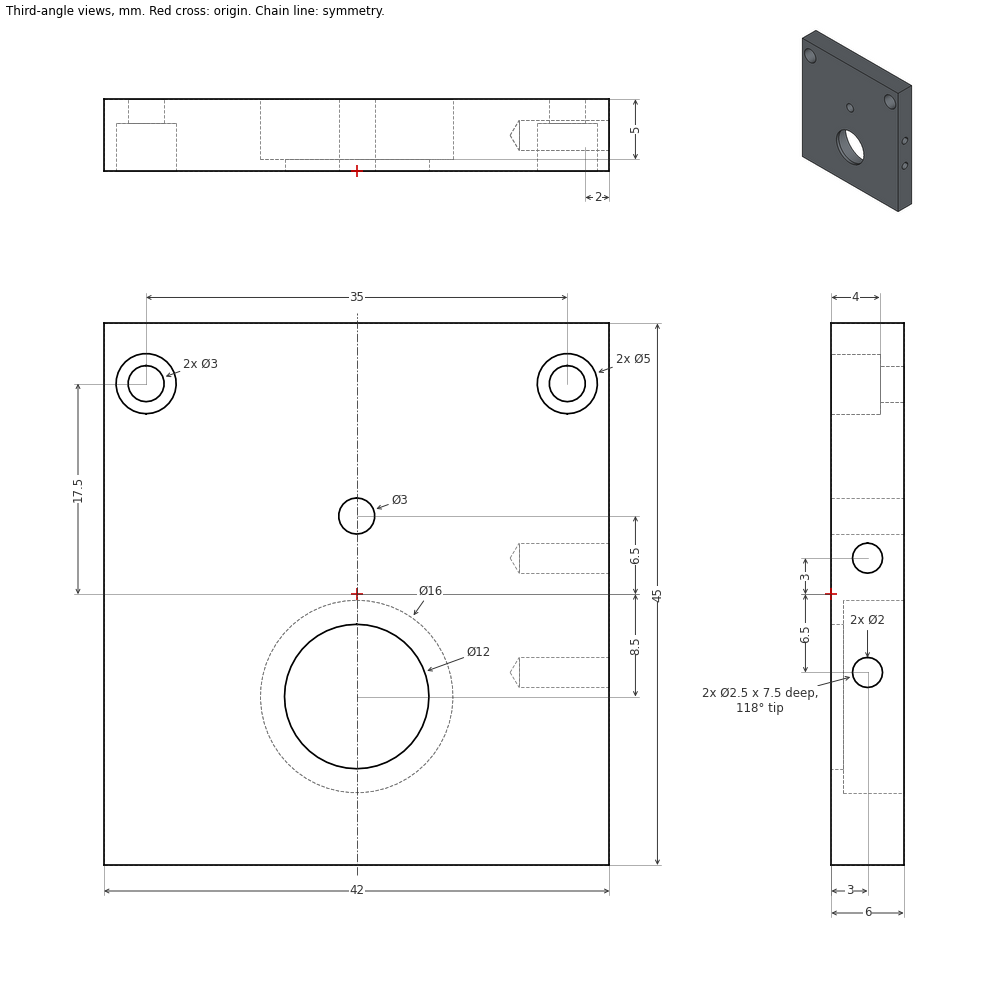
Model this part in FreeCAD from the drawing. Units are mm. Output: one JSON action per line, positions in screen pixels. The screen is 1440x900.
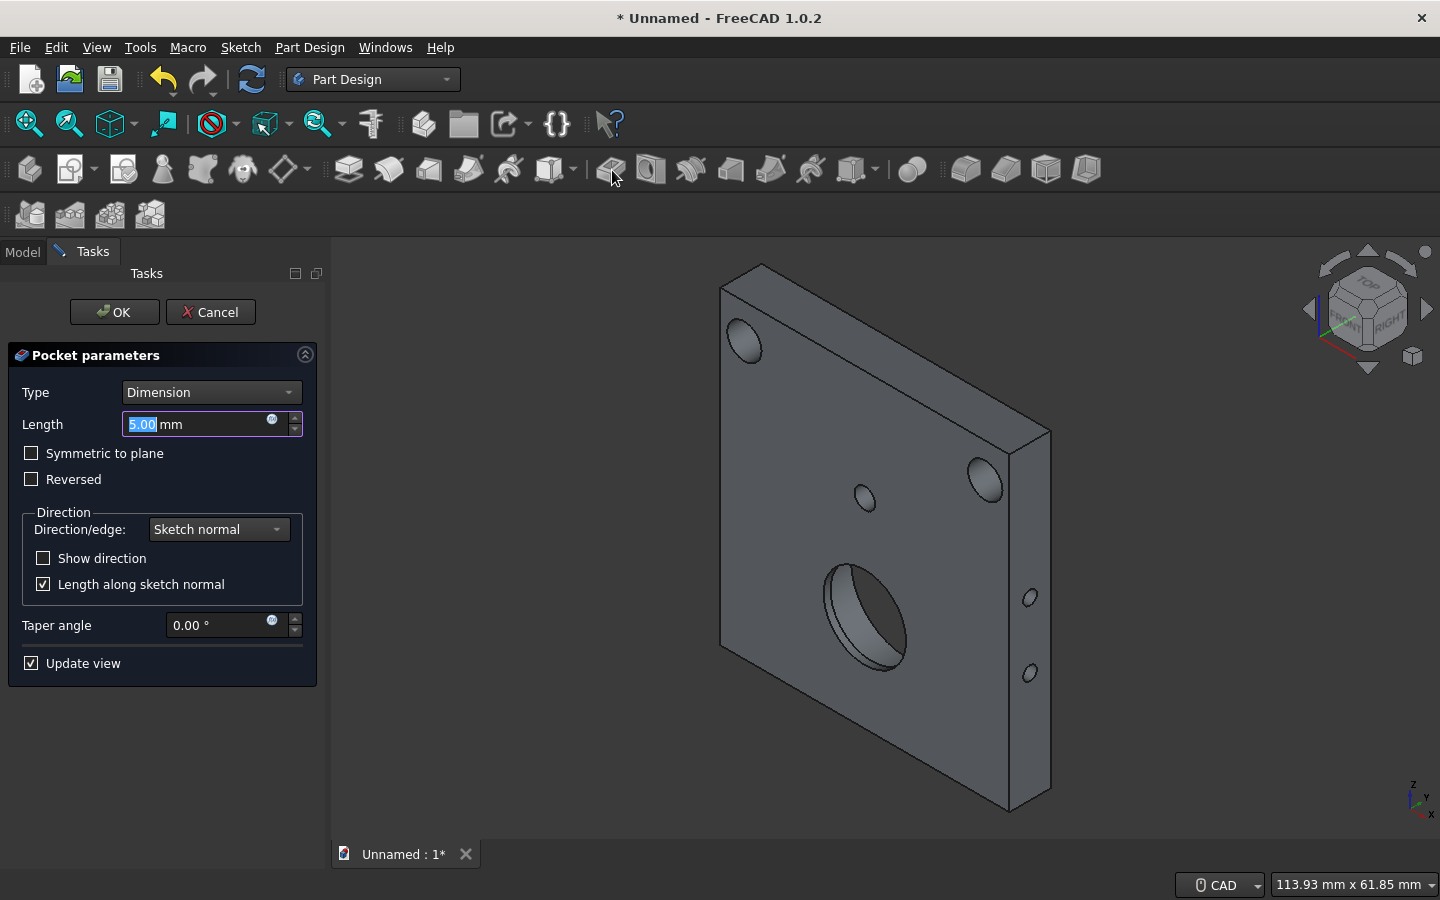
{"action": "type", "text": "2"}
{"action": "key", "text": "Tab"}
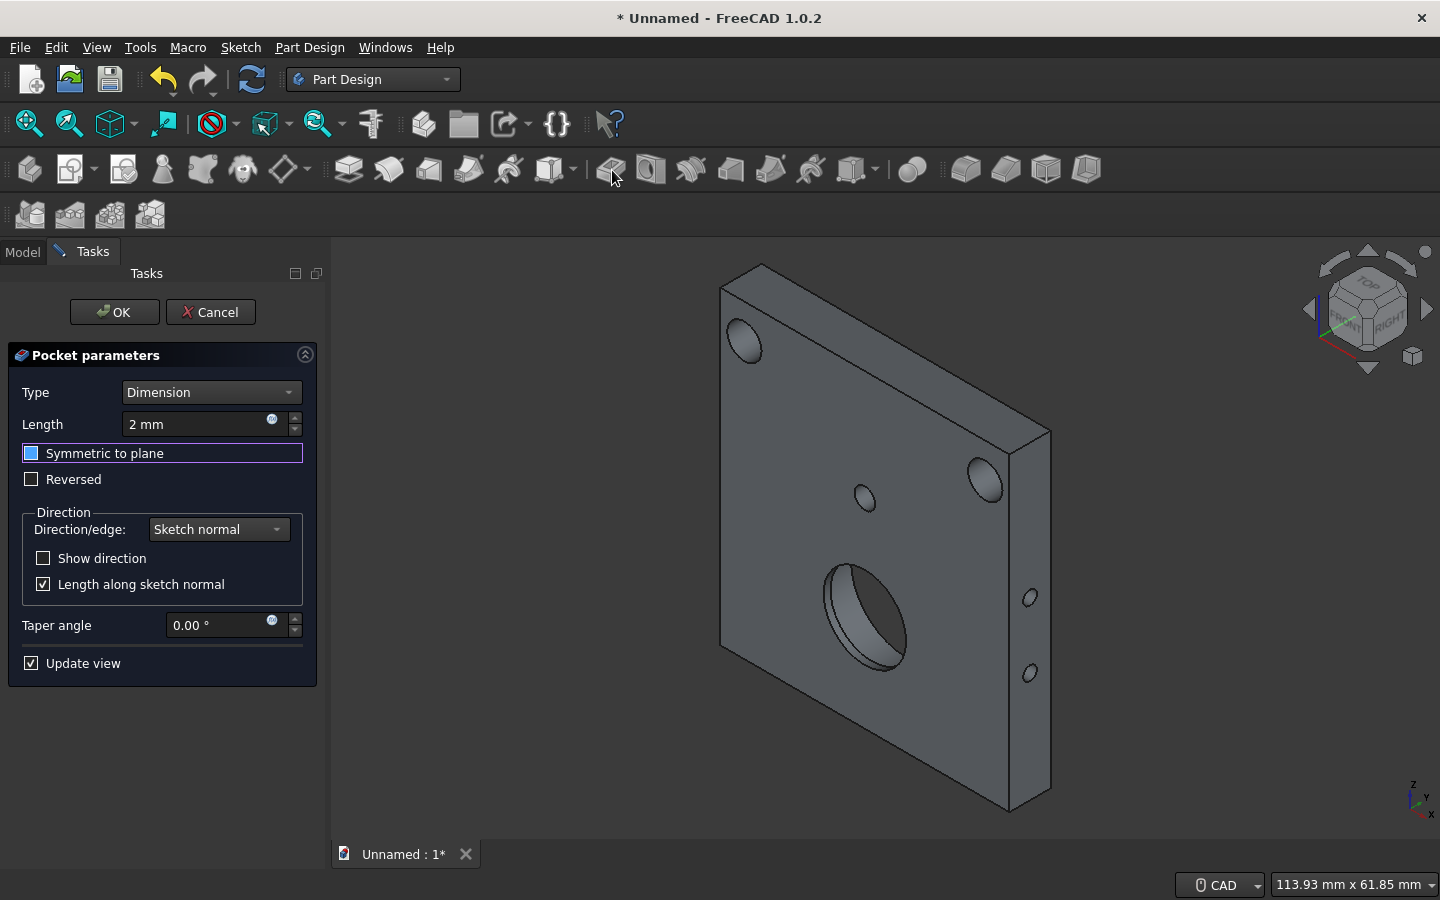
{"action": "left_click", "coordinate": [115, 312]}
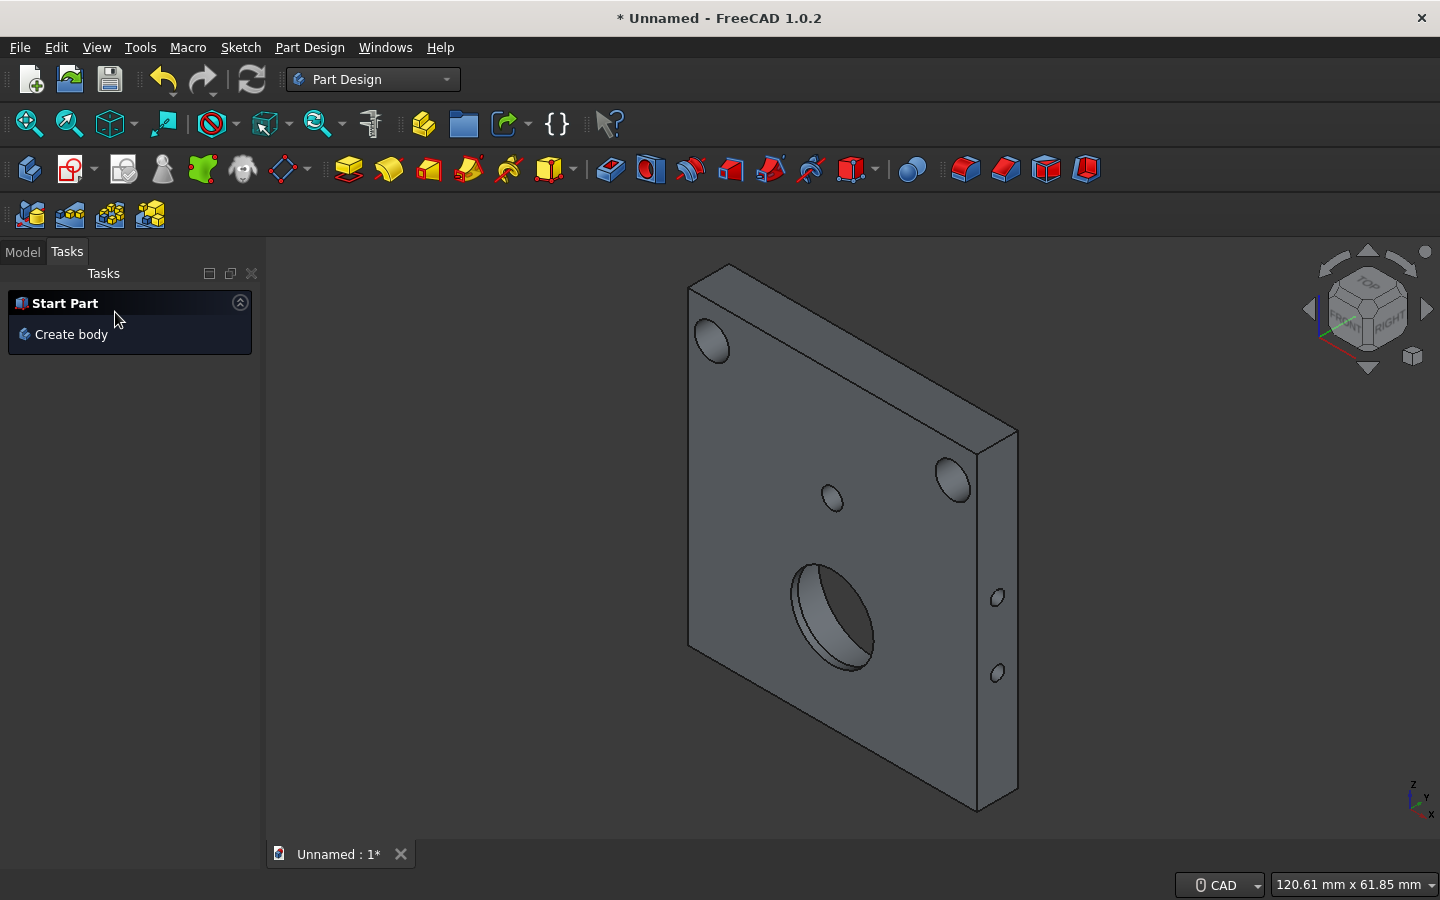
{"action": "left_click", "coordinate": [998, 518]}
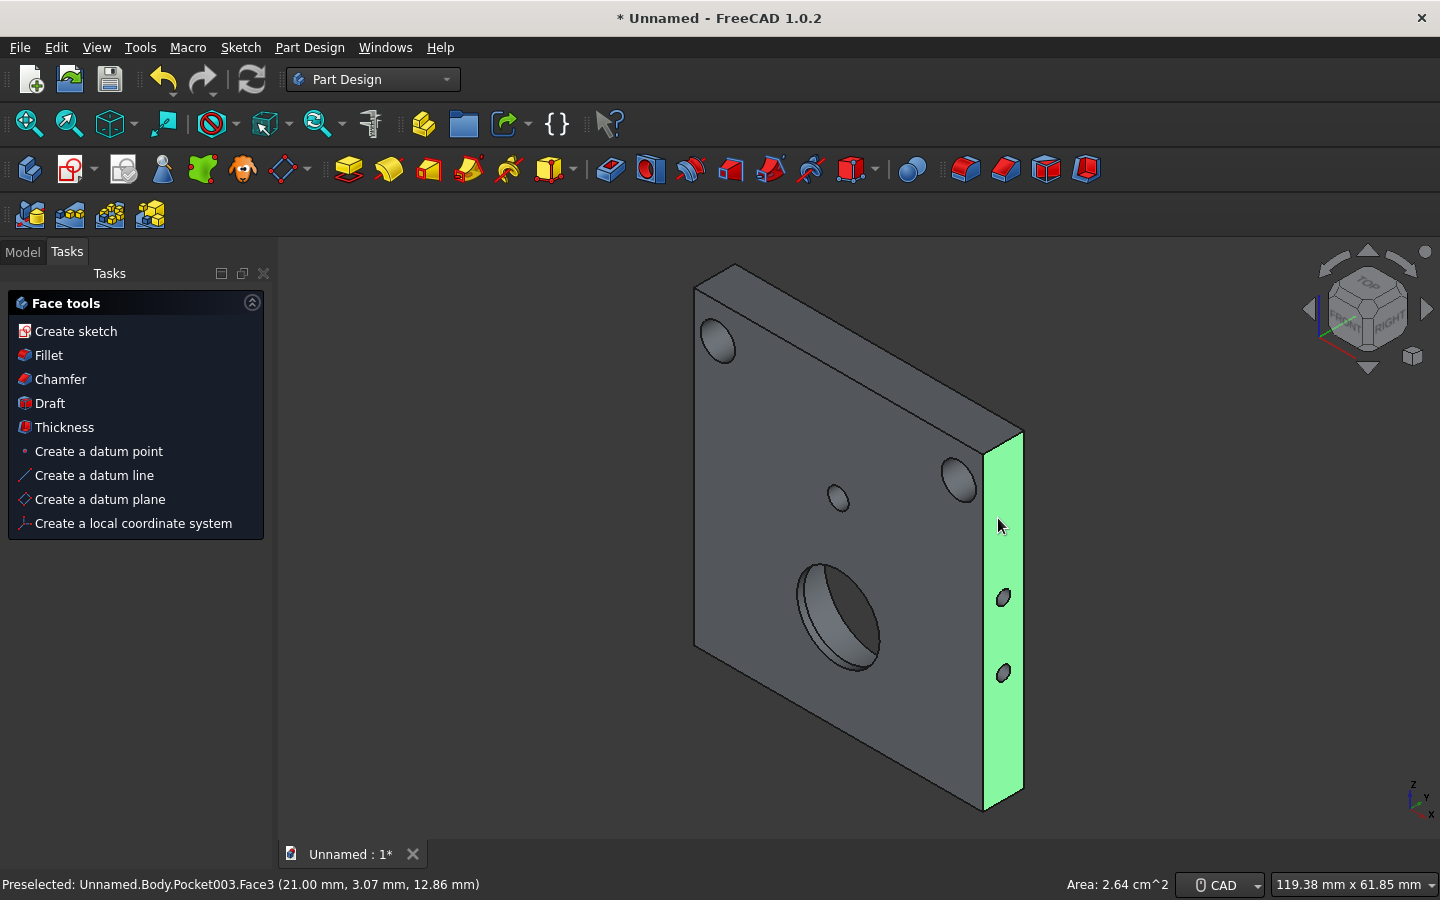
{"action": "left_click", "coordinate": [70, 170]}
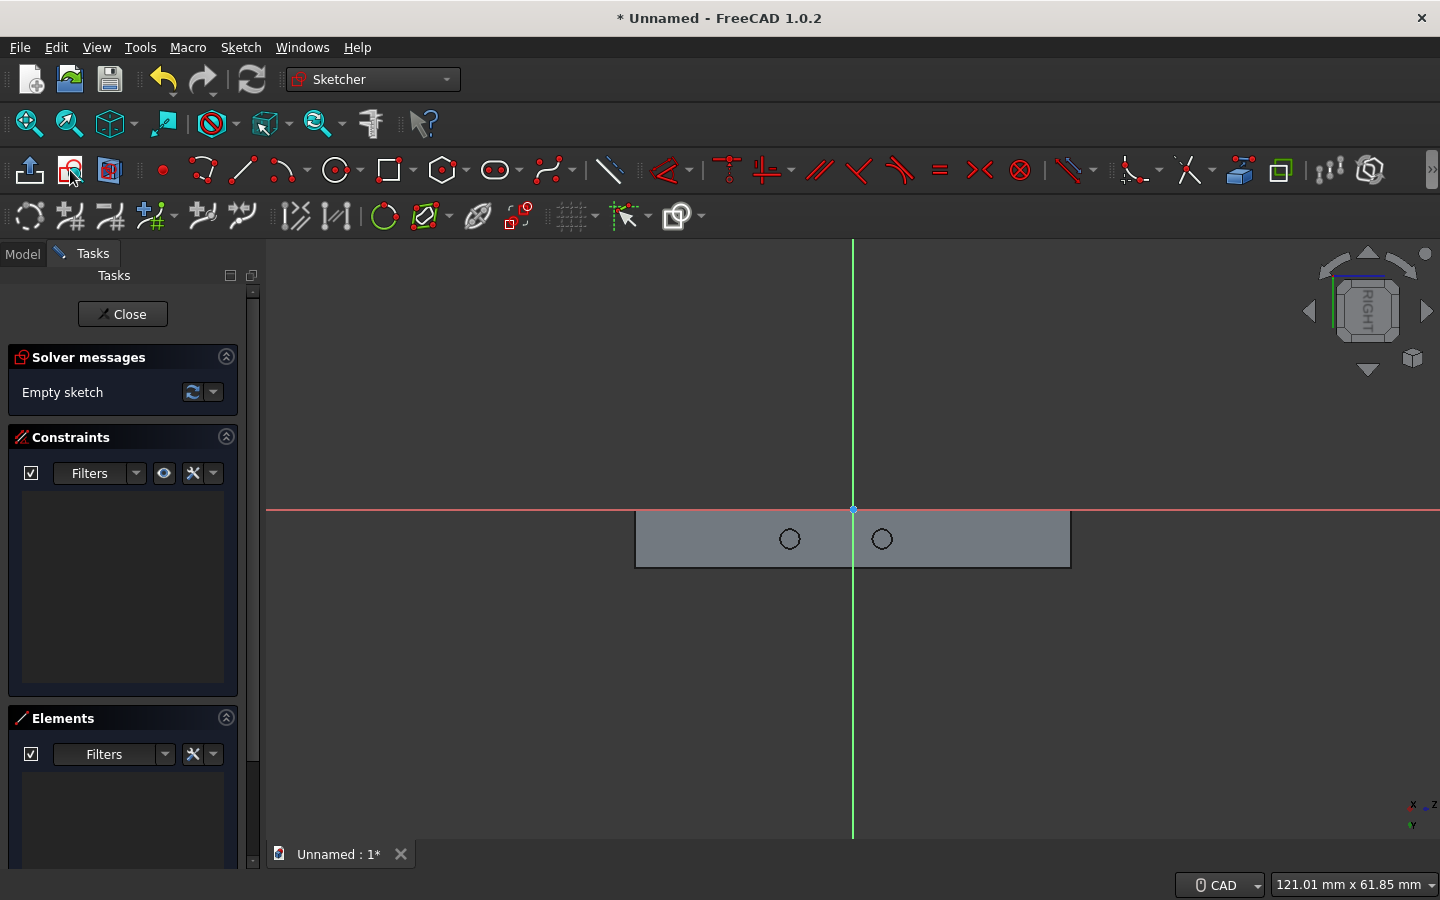
{"action": "scroll", "coordinate": [846, 529], "scroll_direction": "up", "scroll_amount": 9}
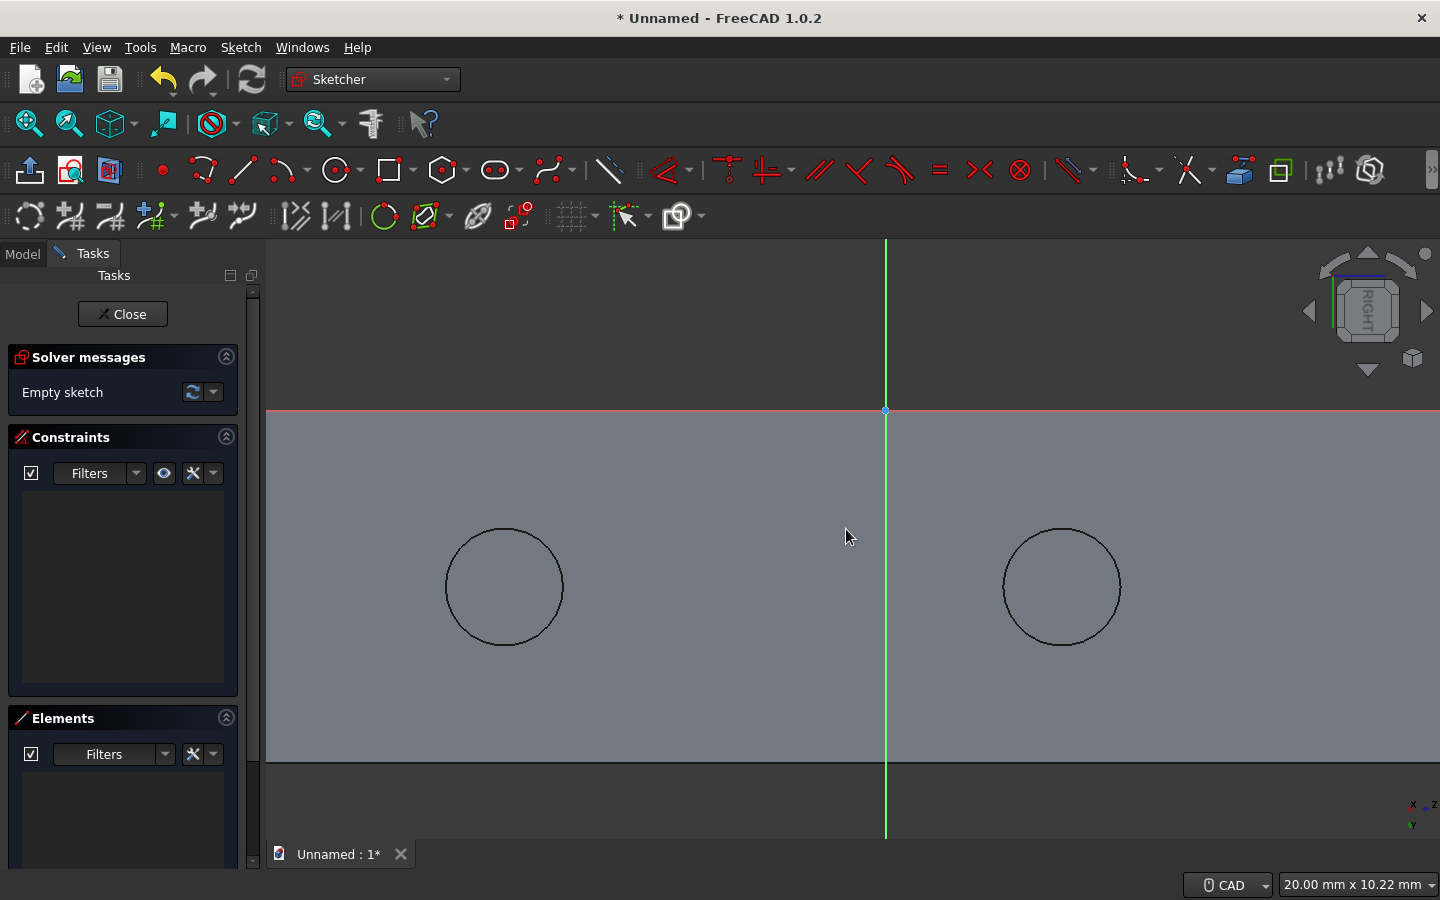
{"action": "key", "text": "g c"}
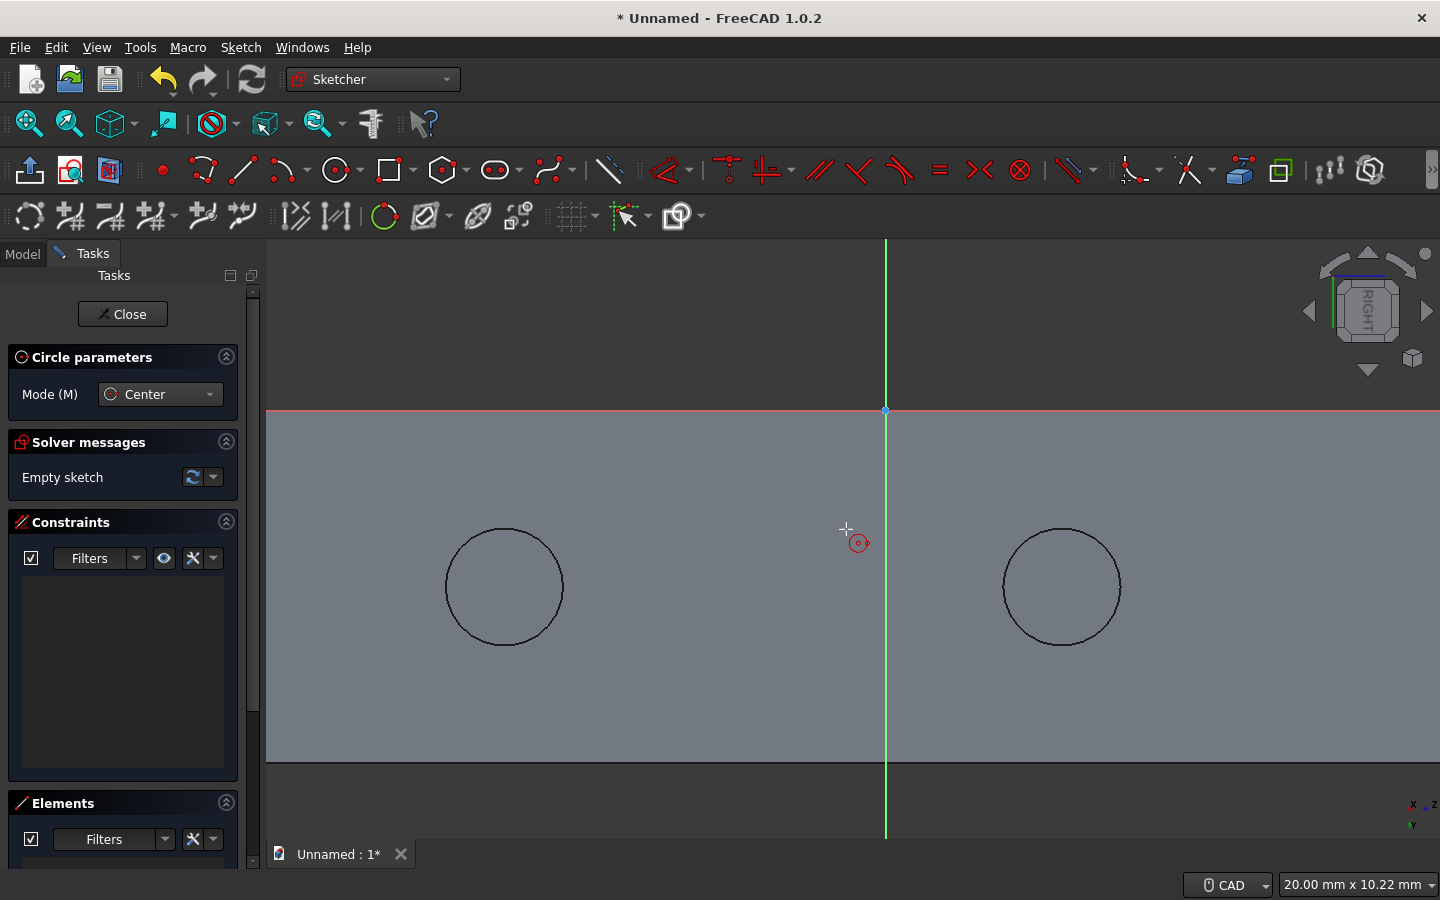
{"action": "left_click", "coordinate": [504, 587]}
{"action": "mouse_move", "coordinate": [556, 535]}